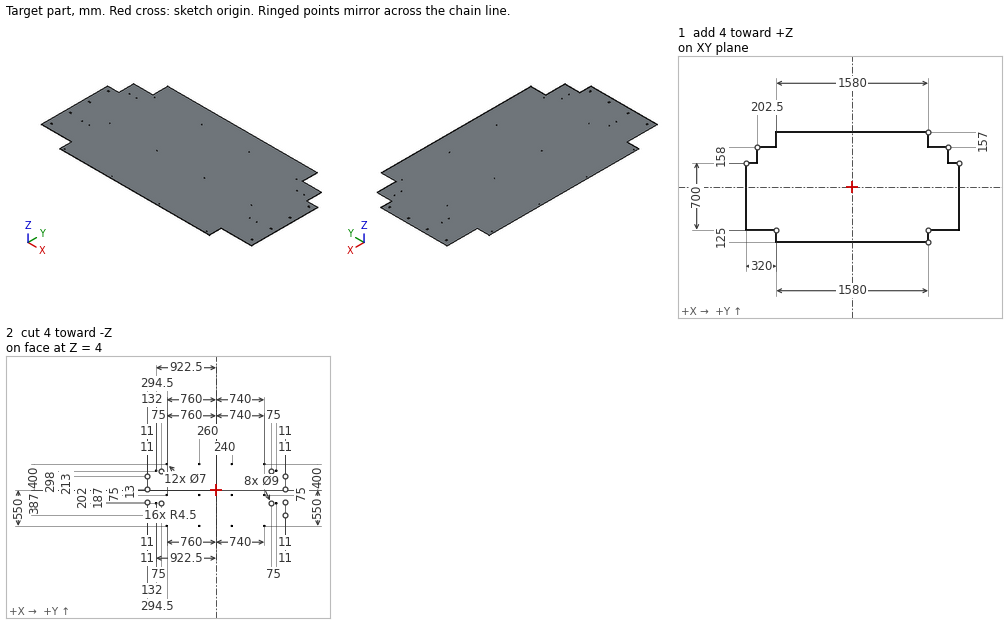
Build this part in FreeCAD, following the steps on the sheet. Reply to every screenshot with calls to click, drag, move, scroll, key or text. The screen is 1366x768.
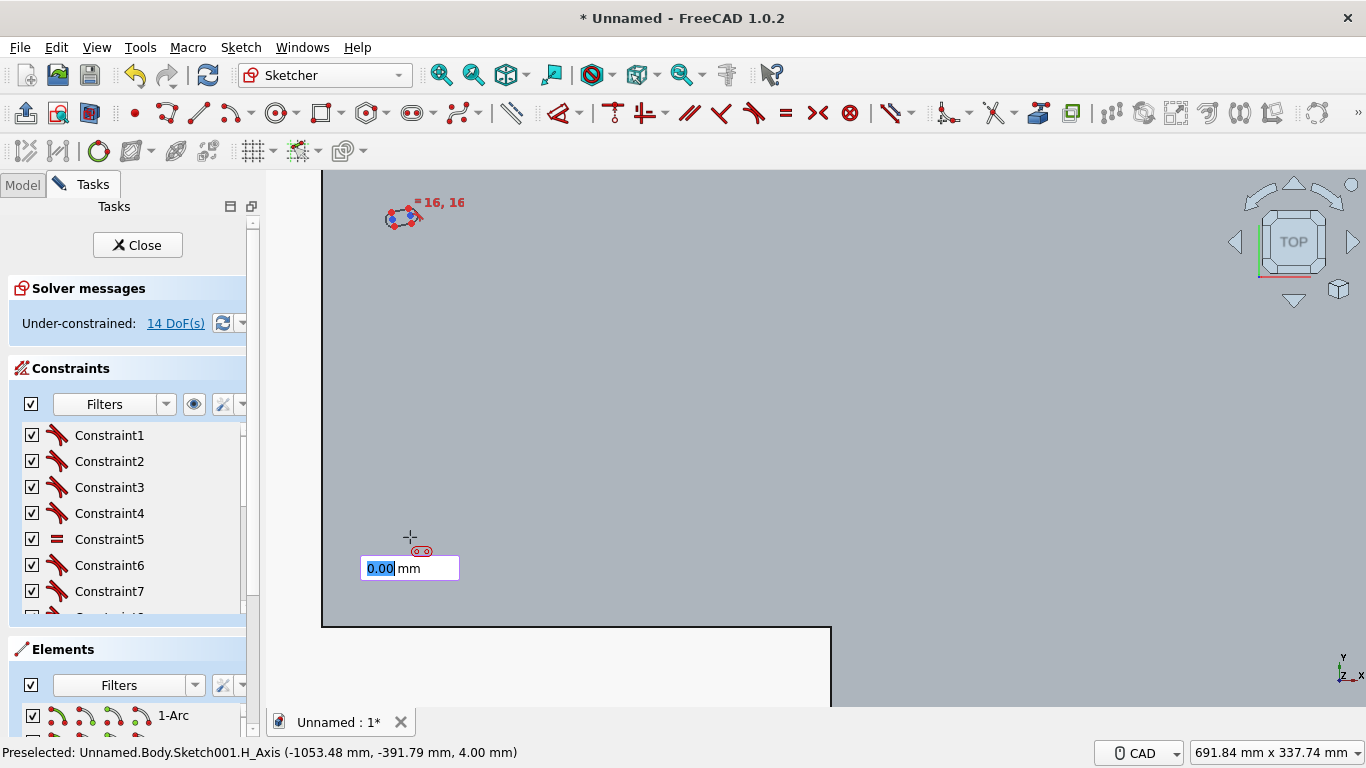
scroll(401, 528, up, 4)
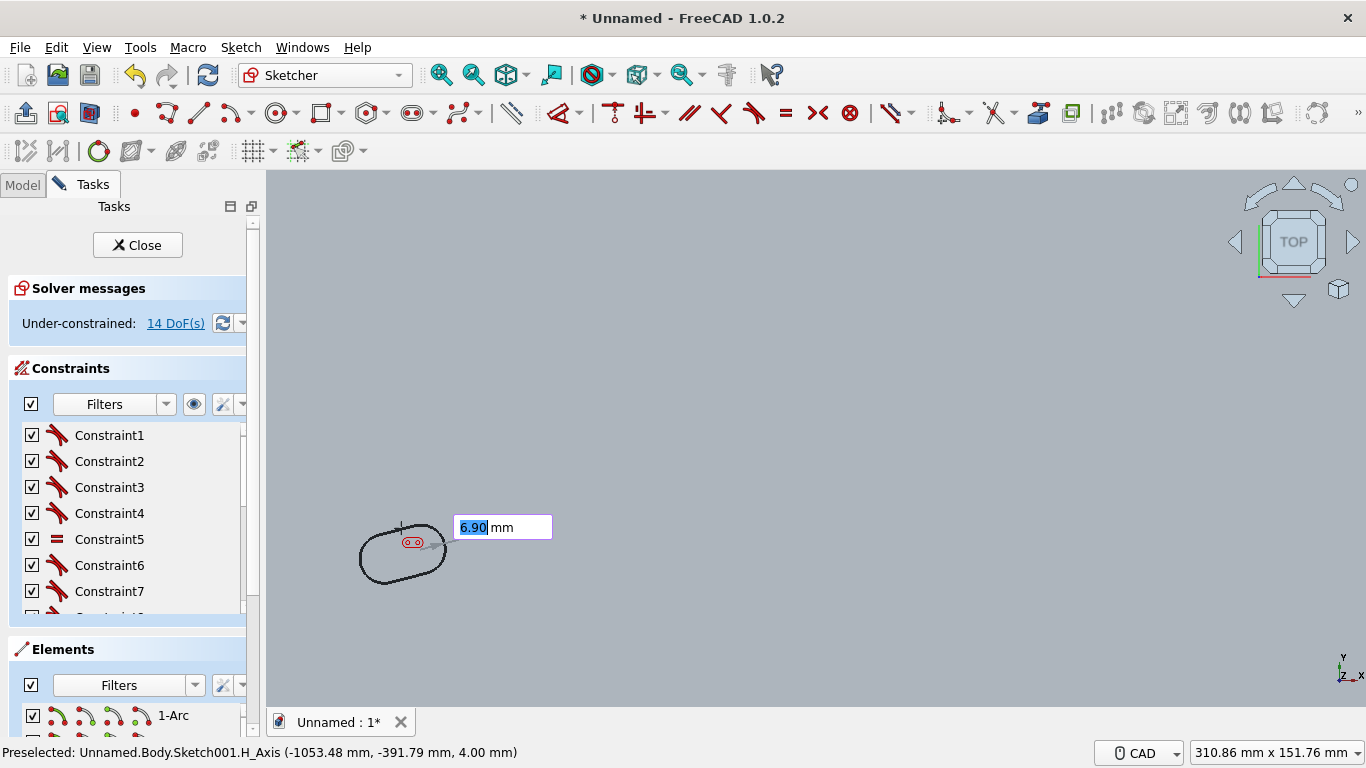
click(401, 527)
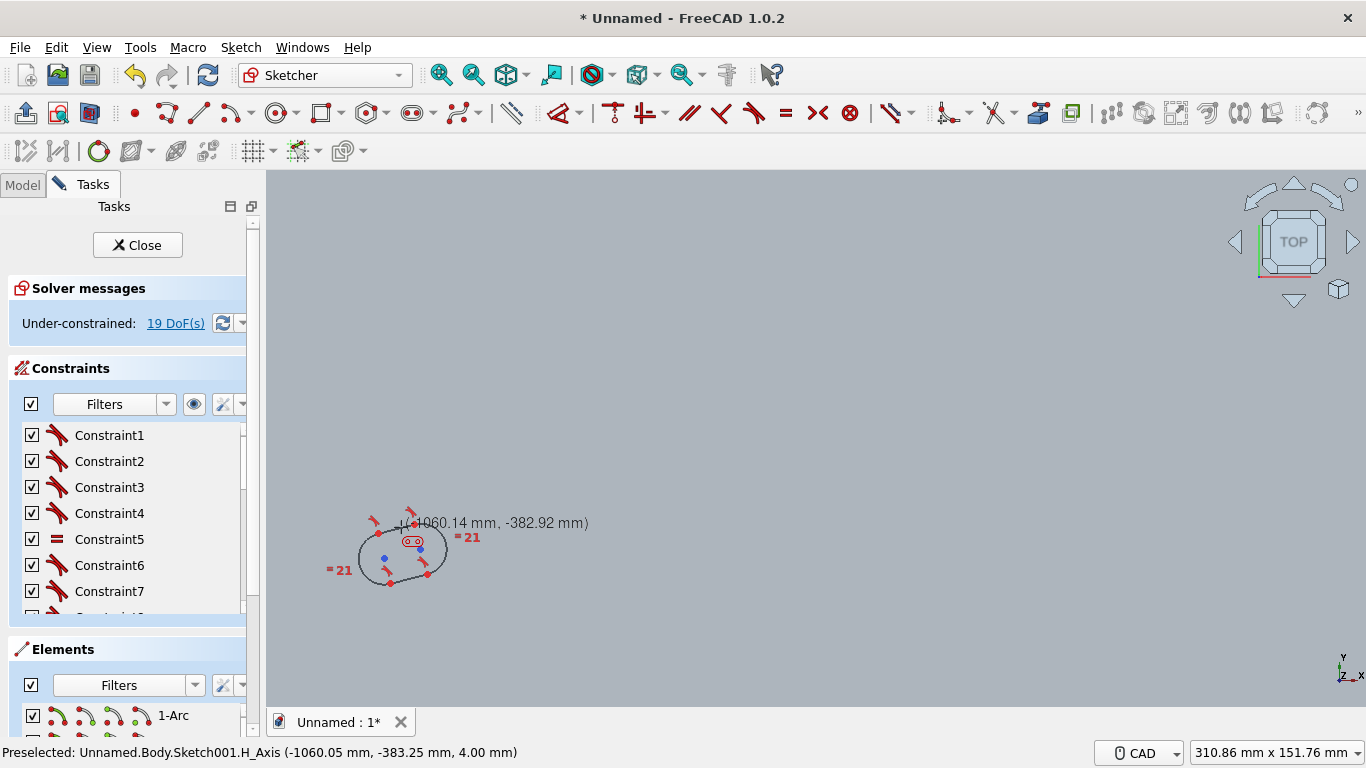
scroll(408, 538, down, 12)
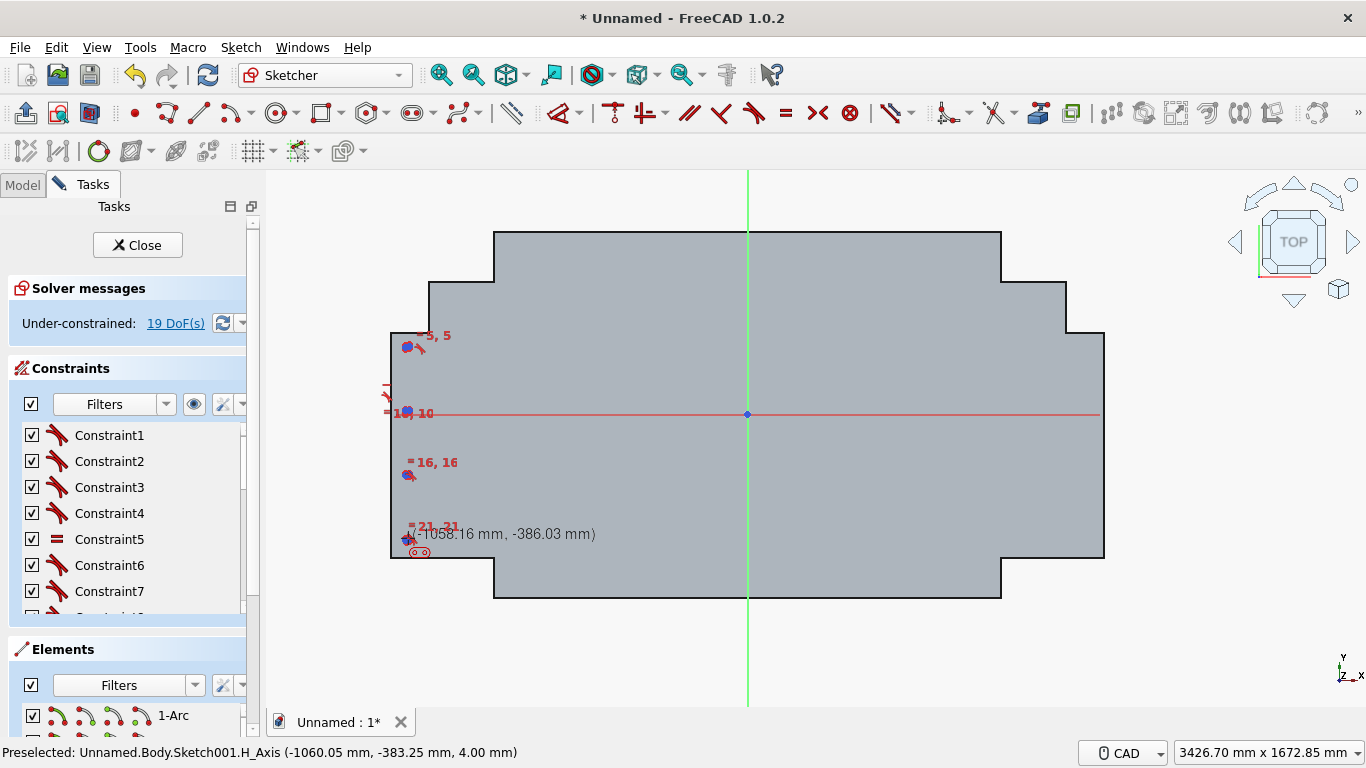
scroll(1086, 539, up, 14)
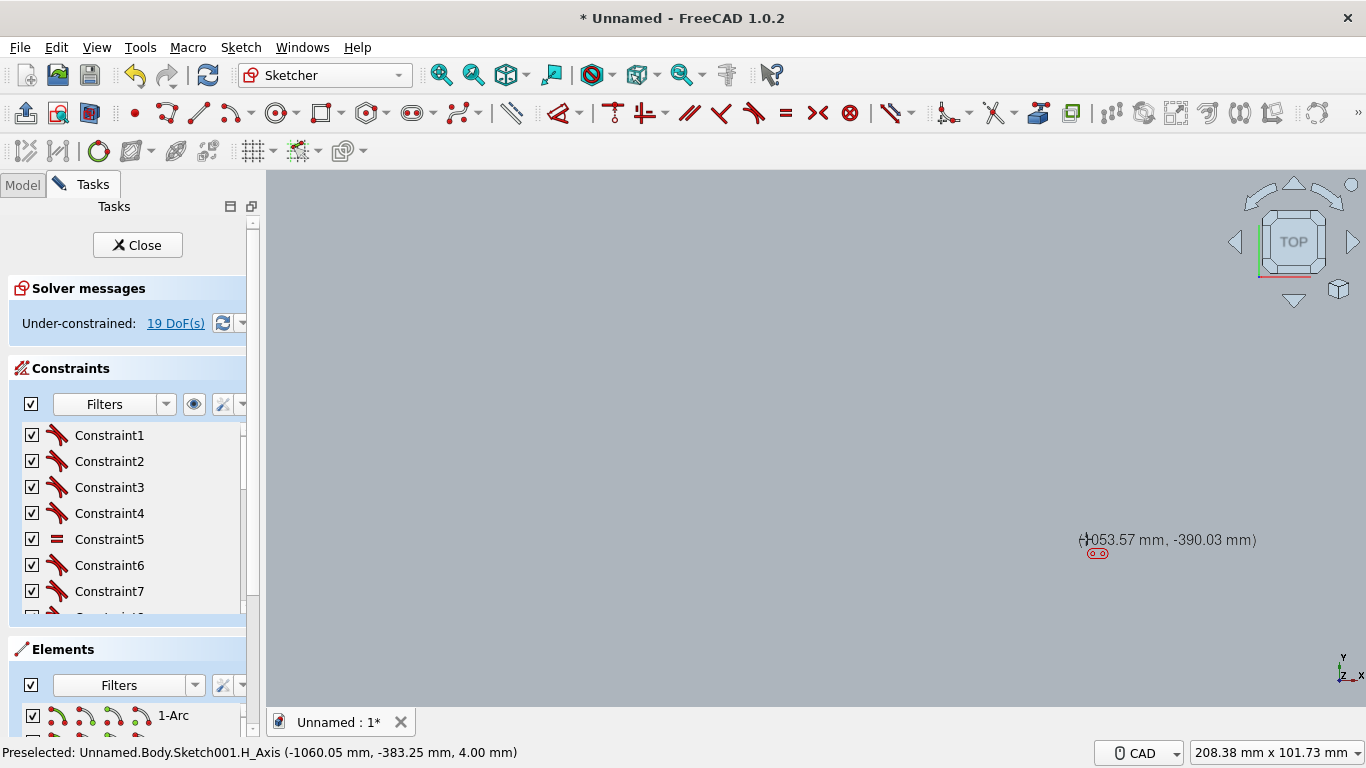
scroll(1086, 539, down, 14)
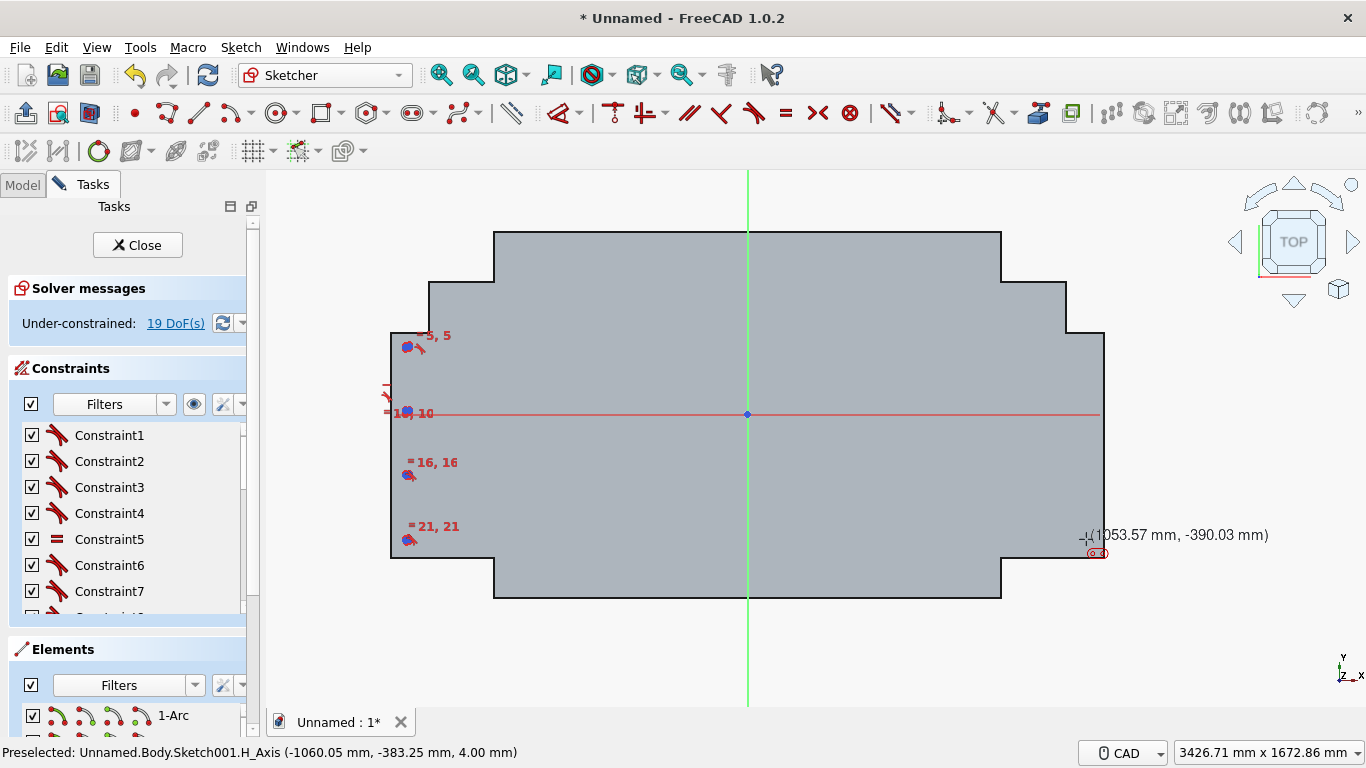
click(1086, 539)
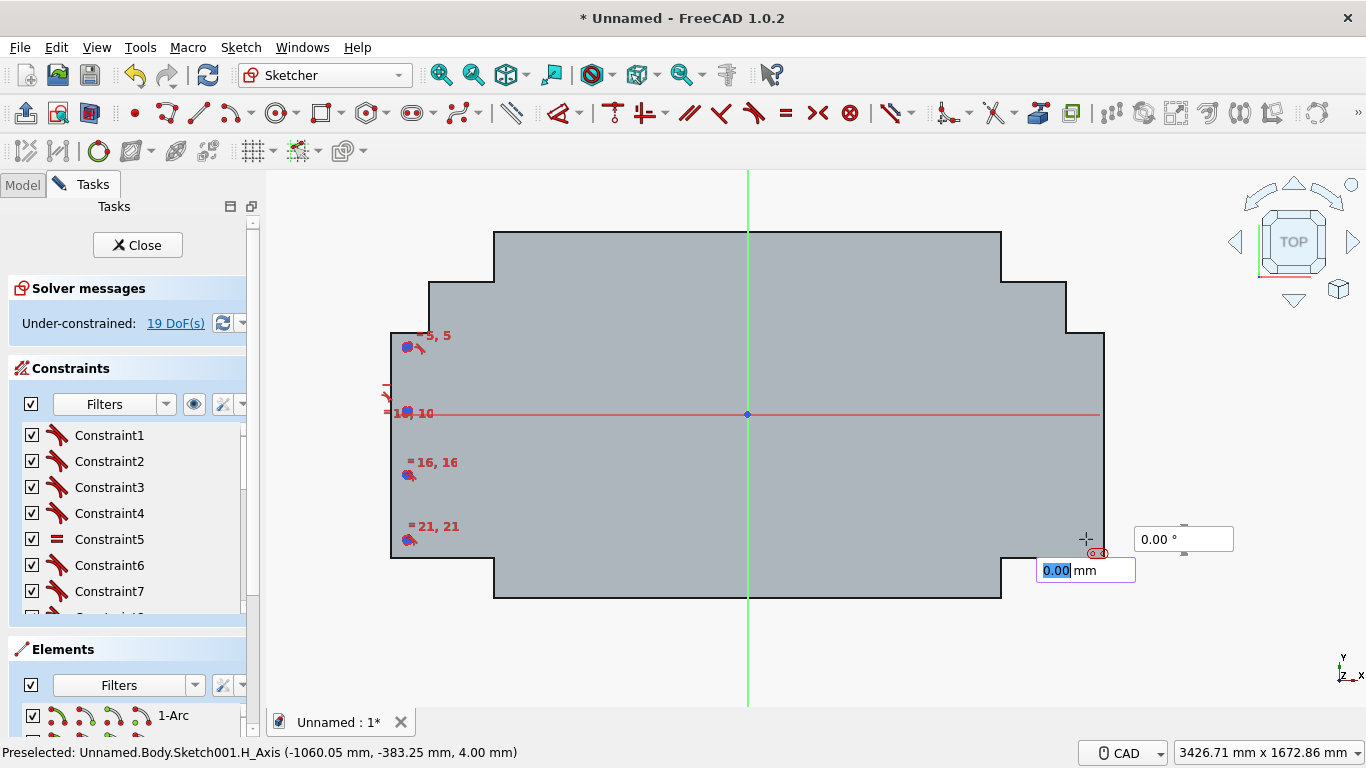
scroll(1090, 539, up, 8)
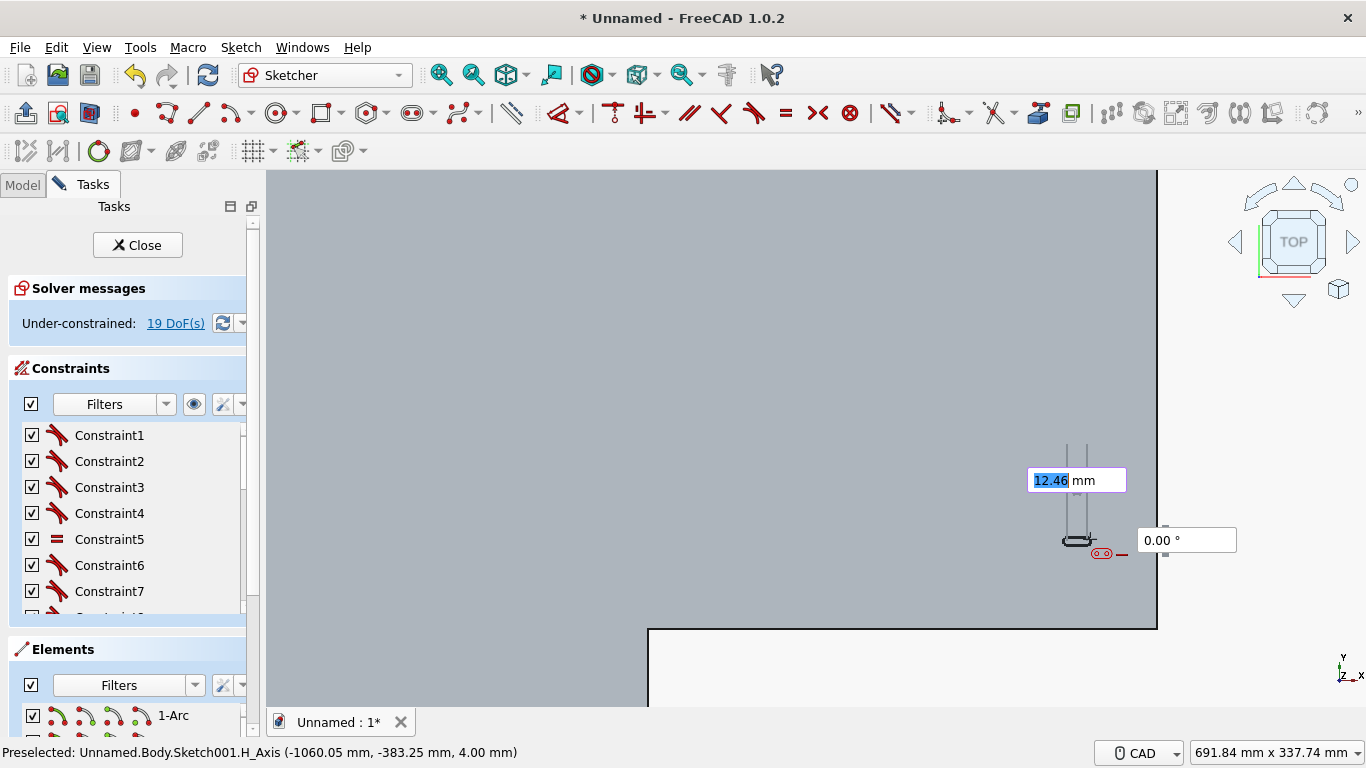
click(1086, 536)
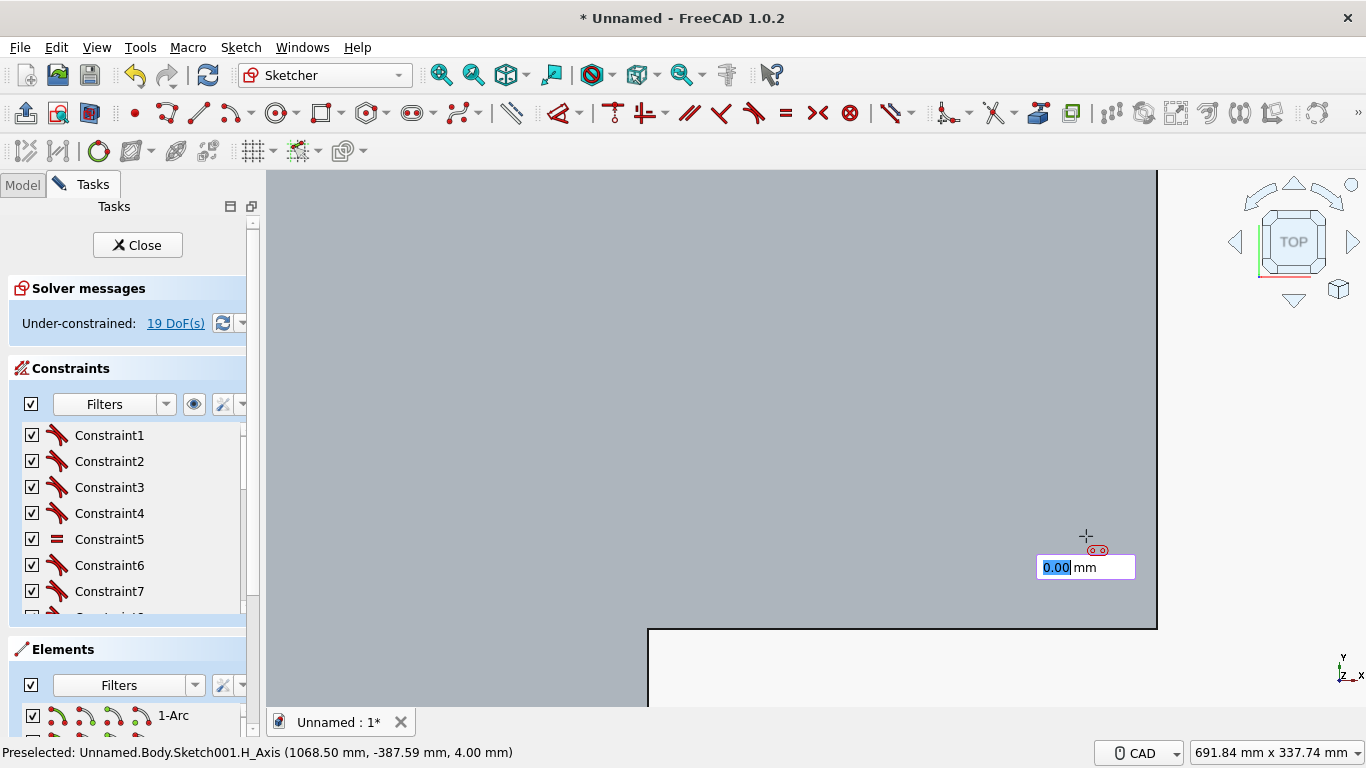
scroll(1077, 529, up, 4)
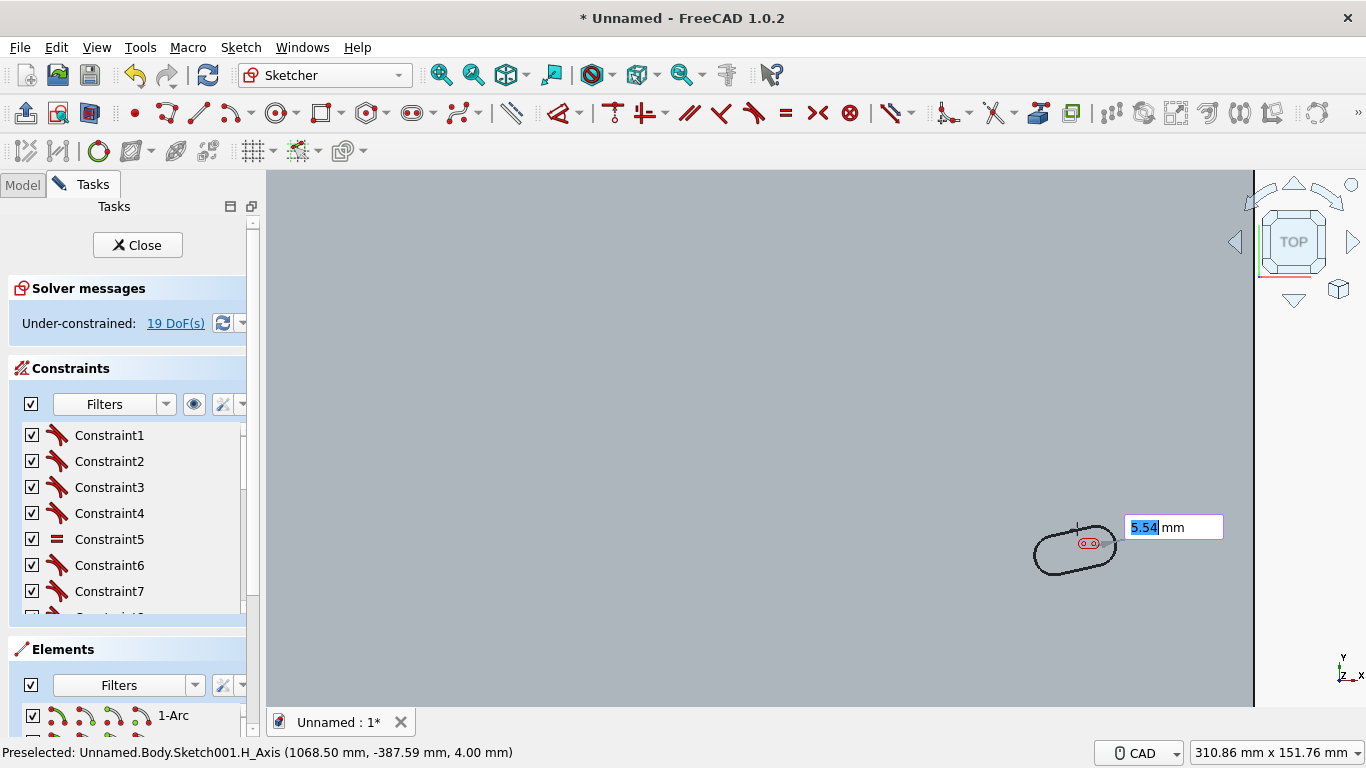
click(1077, 529)